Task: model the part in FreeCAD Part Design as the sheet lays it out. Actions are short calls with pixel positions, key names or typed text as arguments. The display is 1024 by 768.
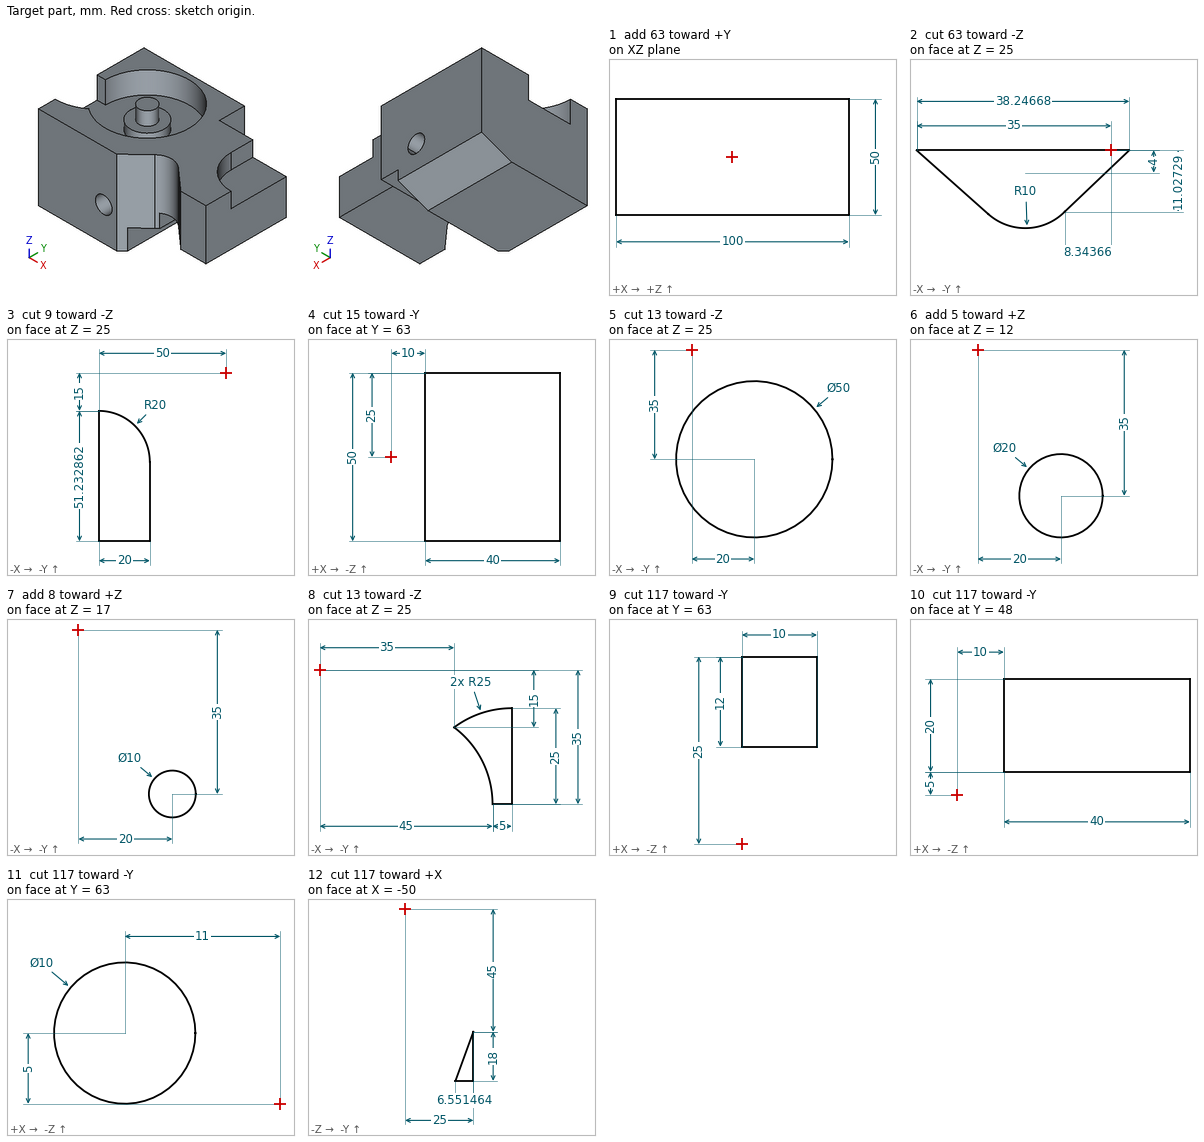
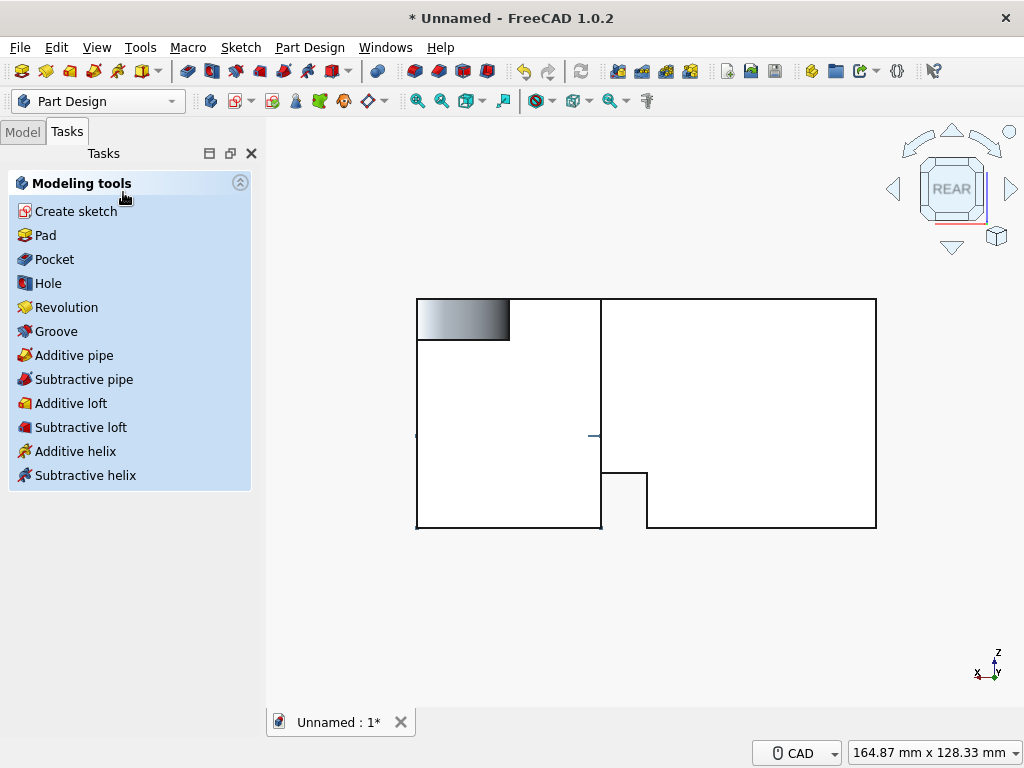
click(188, 72)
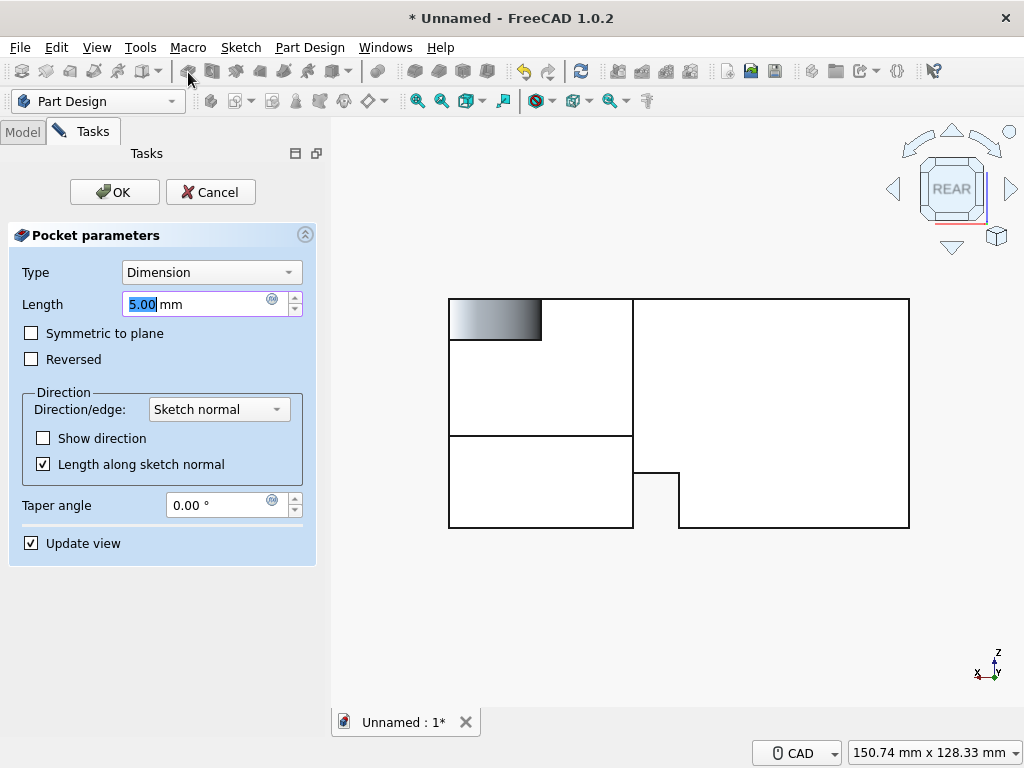
text(117)
key(Tab)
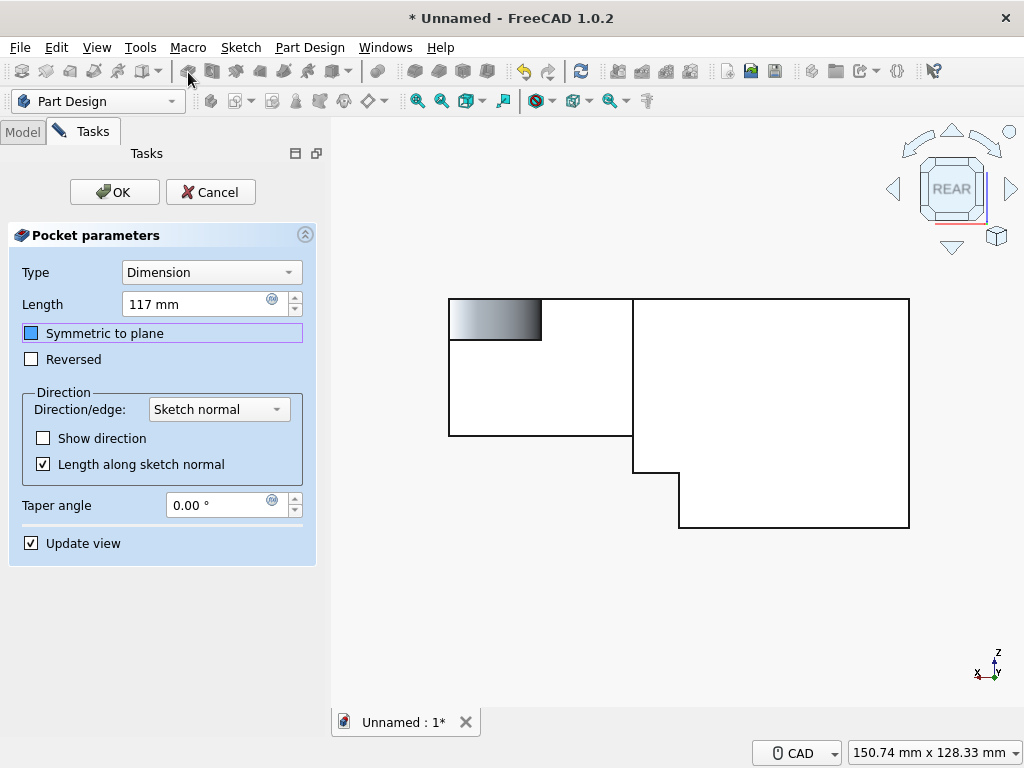
click(115, 192)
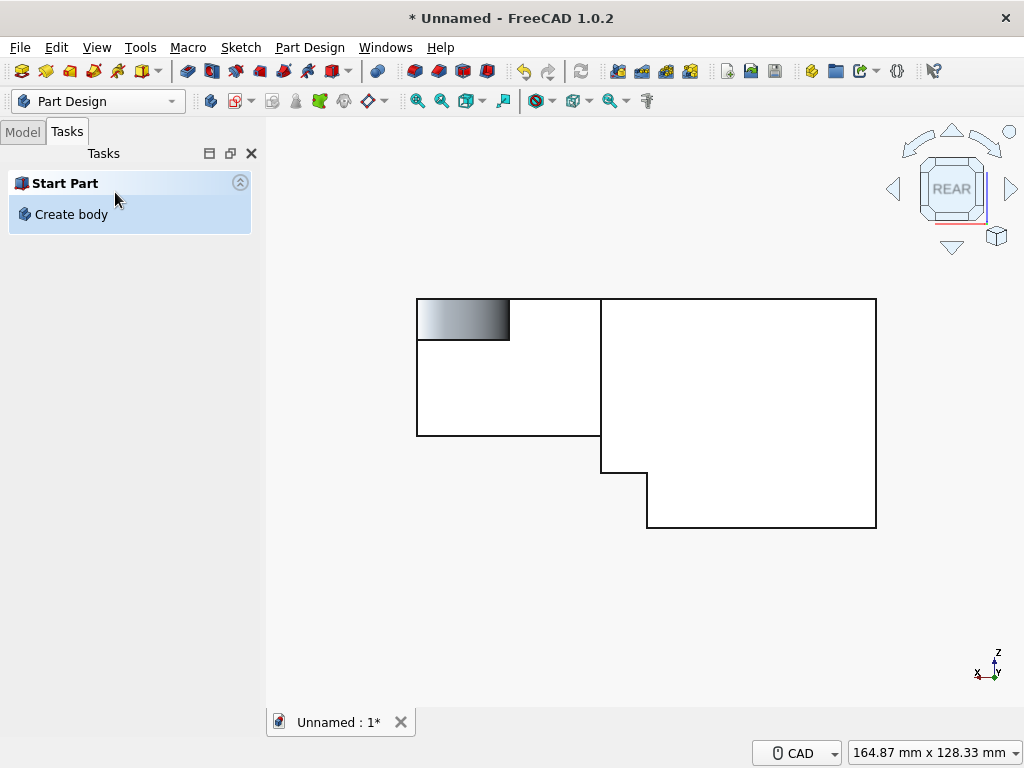
click(738, 412)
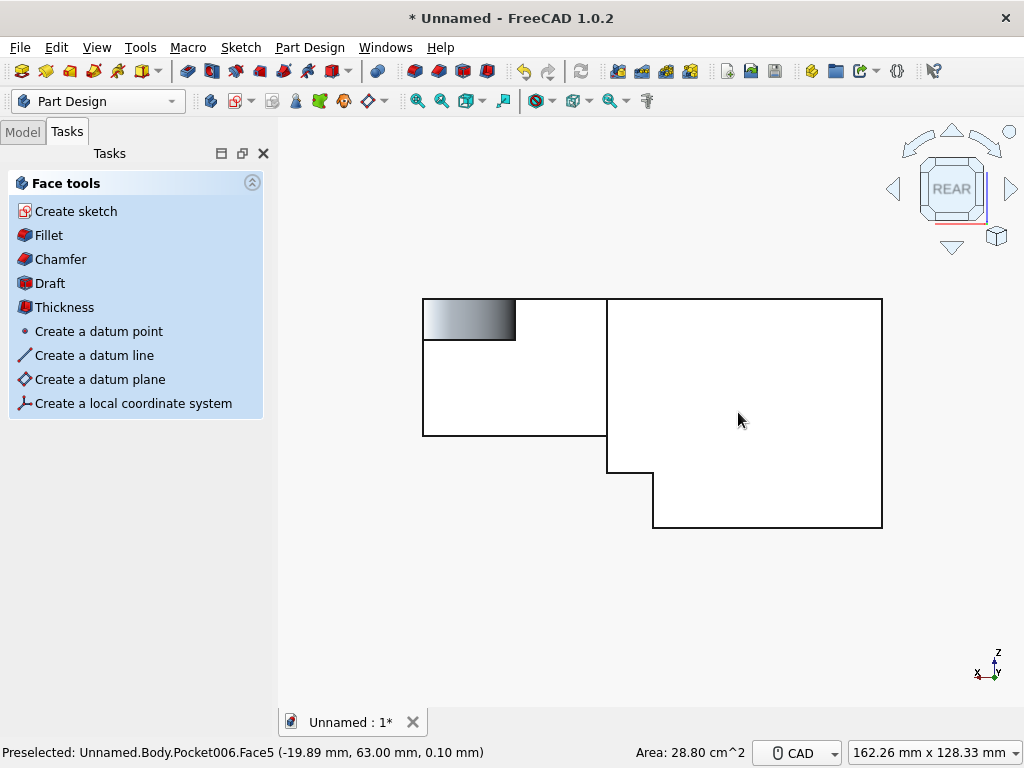
click(236, 102)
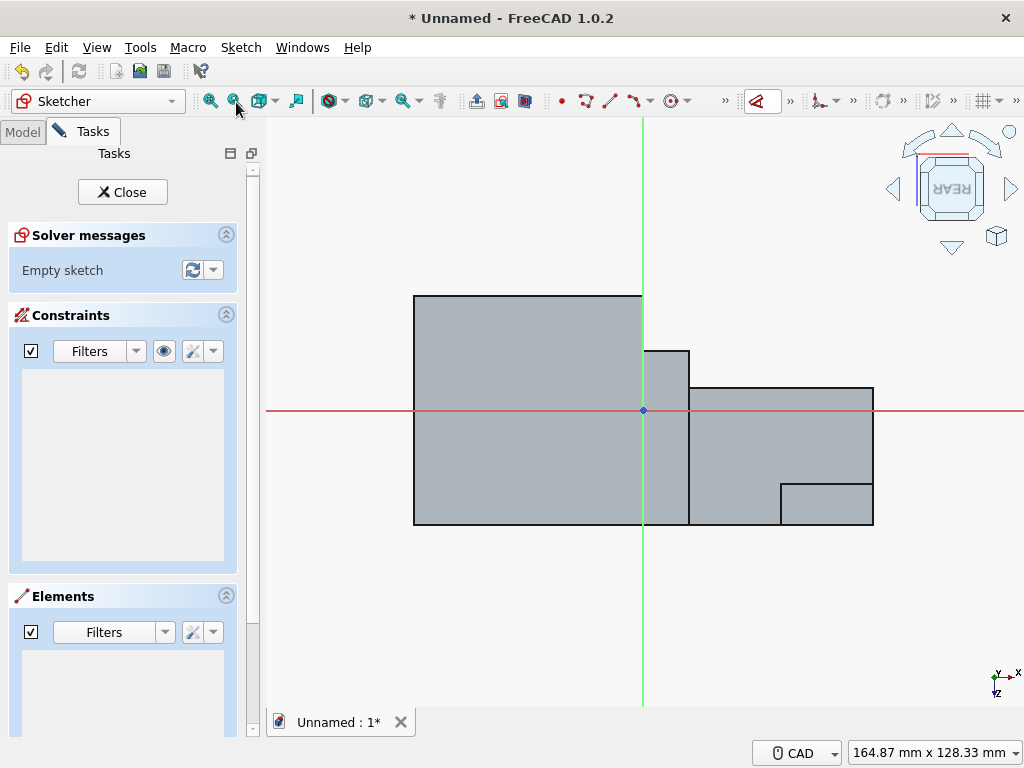
scroll(614, 381, up, 8)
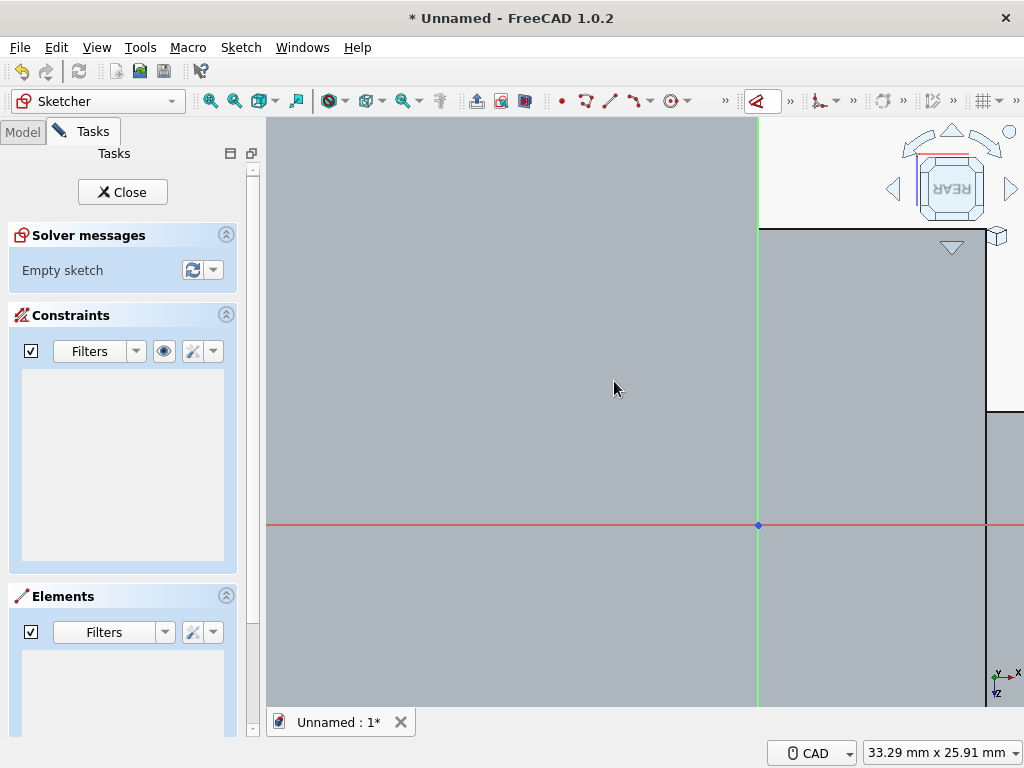
click(672, 102)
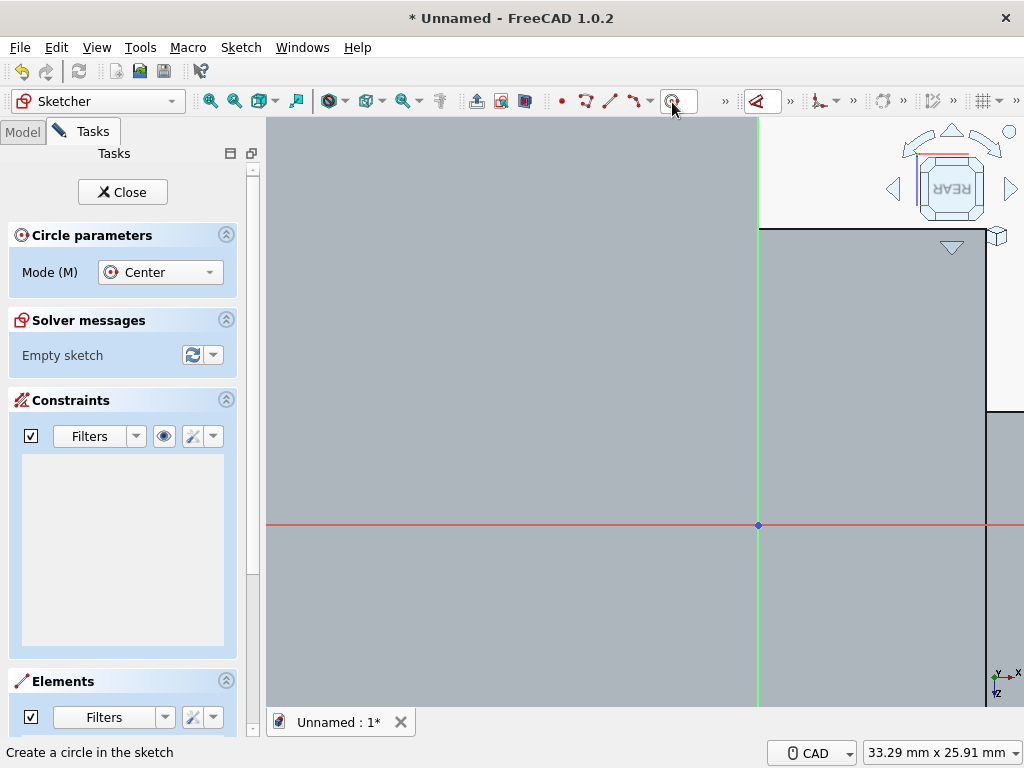
click(508, 412)
click(588, 331)
key(Escape)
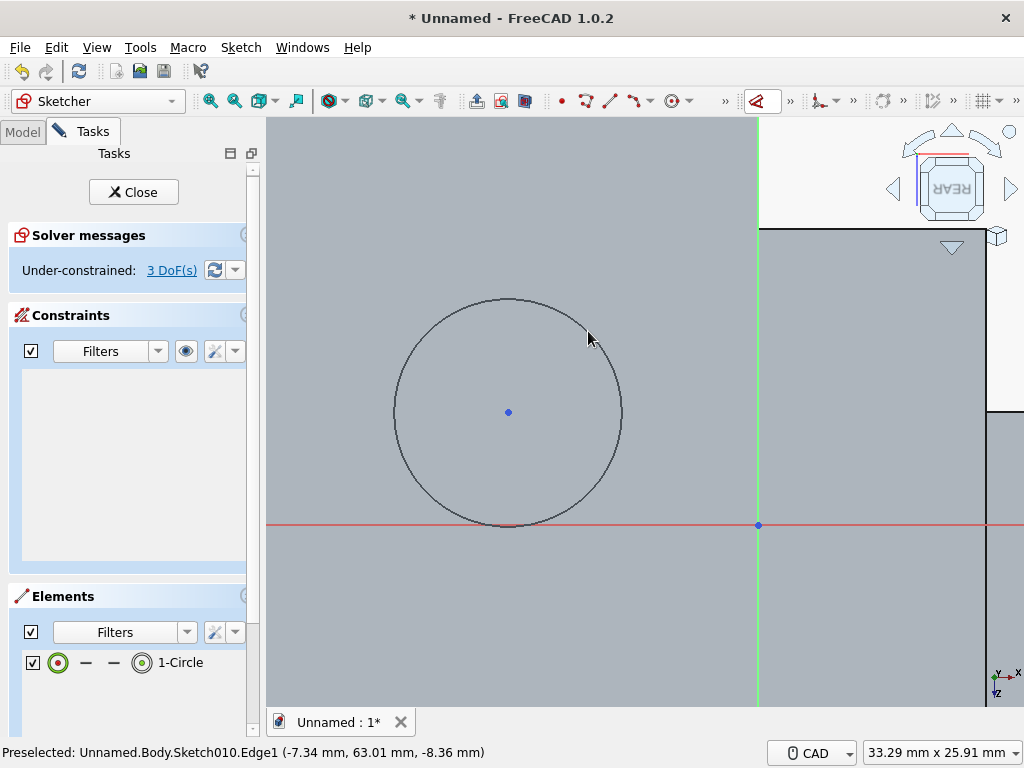
click(588, 332)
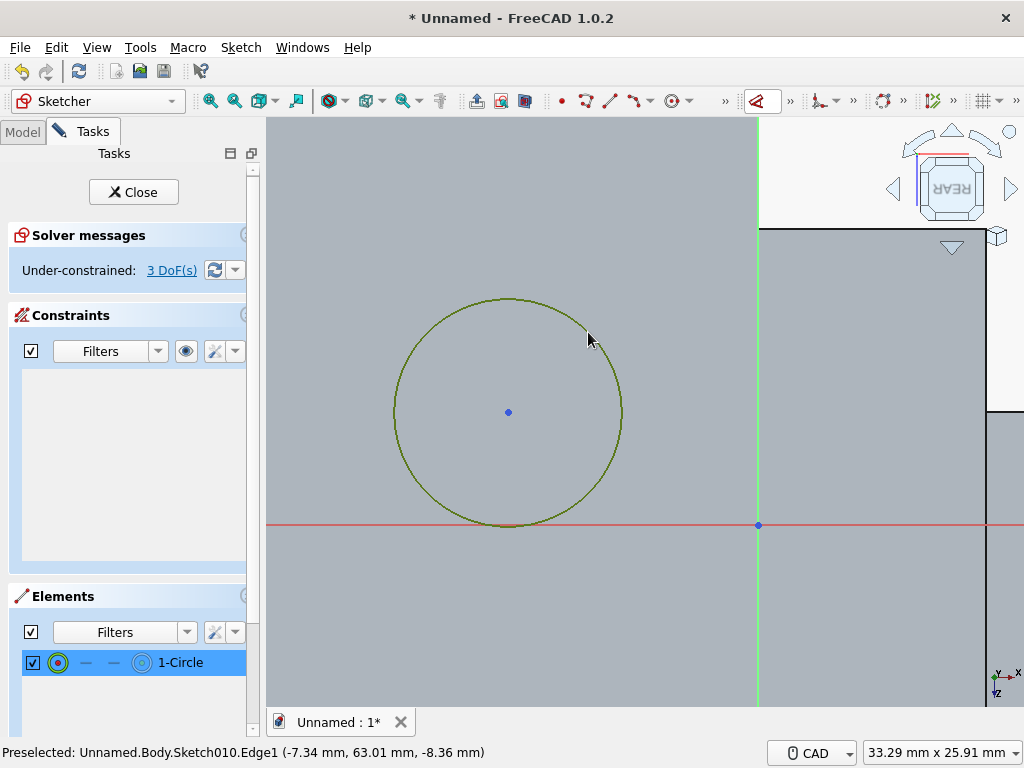
click(776, 102)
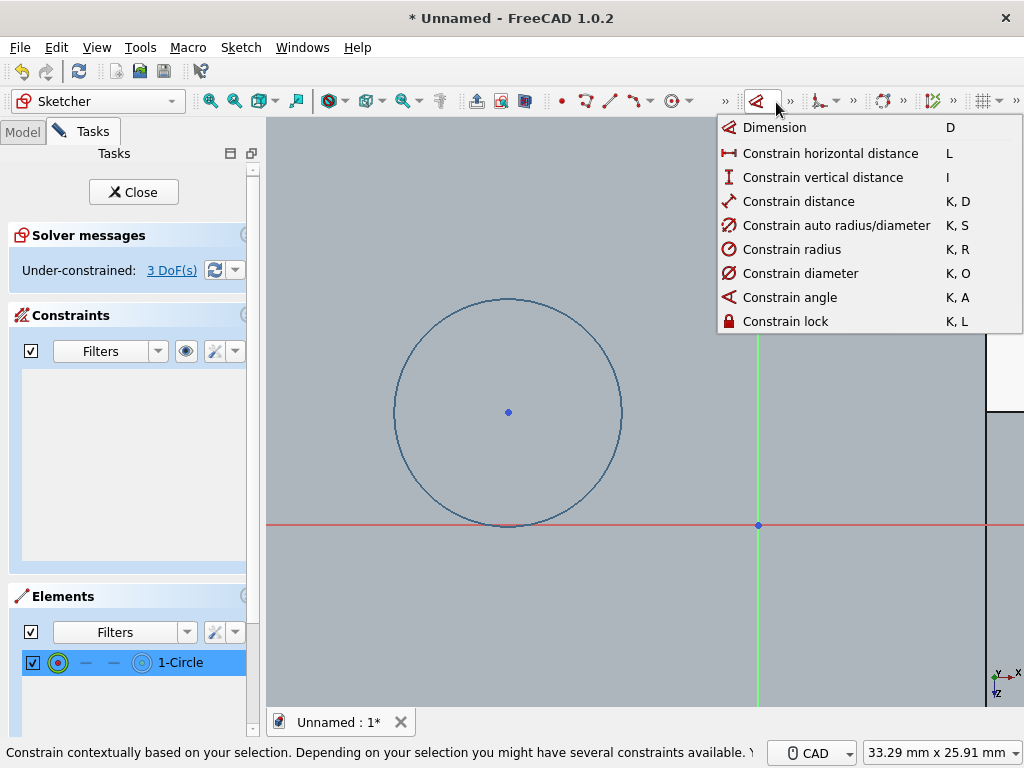
click(870, 273)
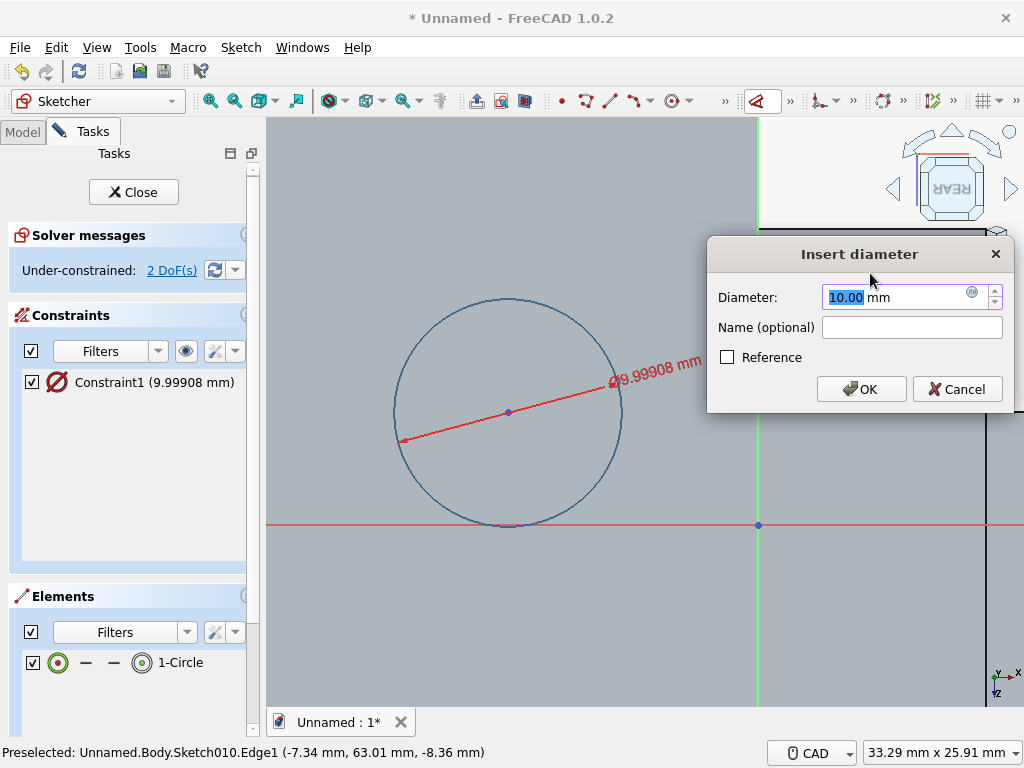
text(10)
key(Return)